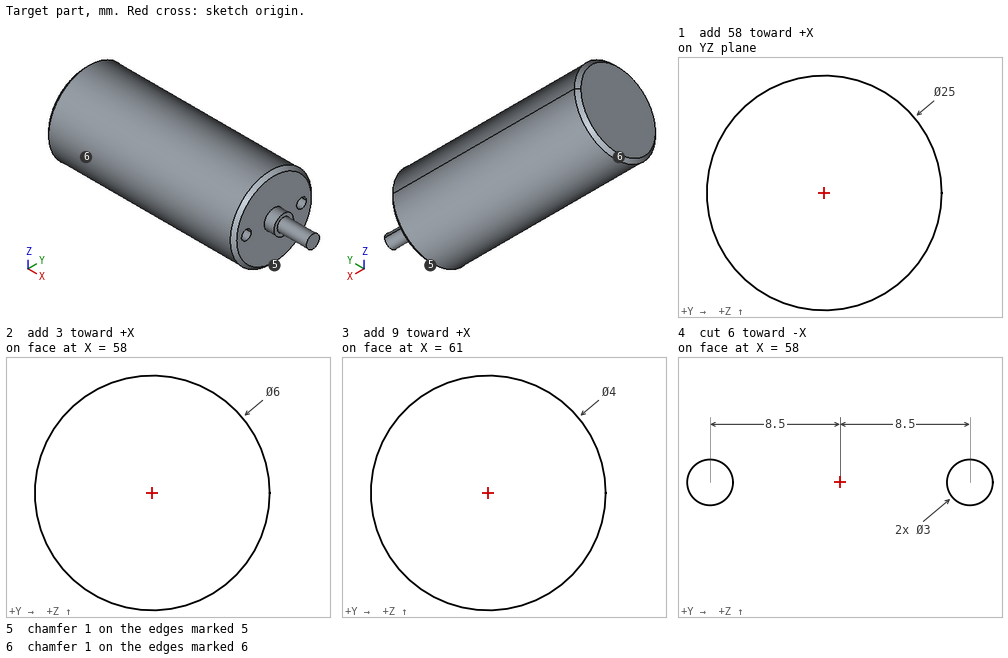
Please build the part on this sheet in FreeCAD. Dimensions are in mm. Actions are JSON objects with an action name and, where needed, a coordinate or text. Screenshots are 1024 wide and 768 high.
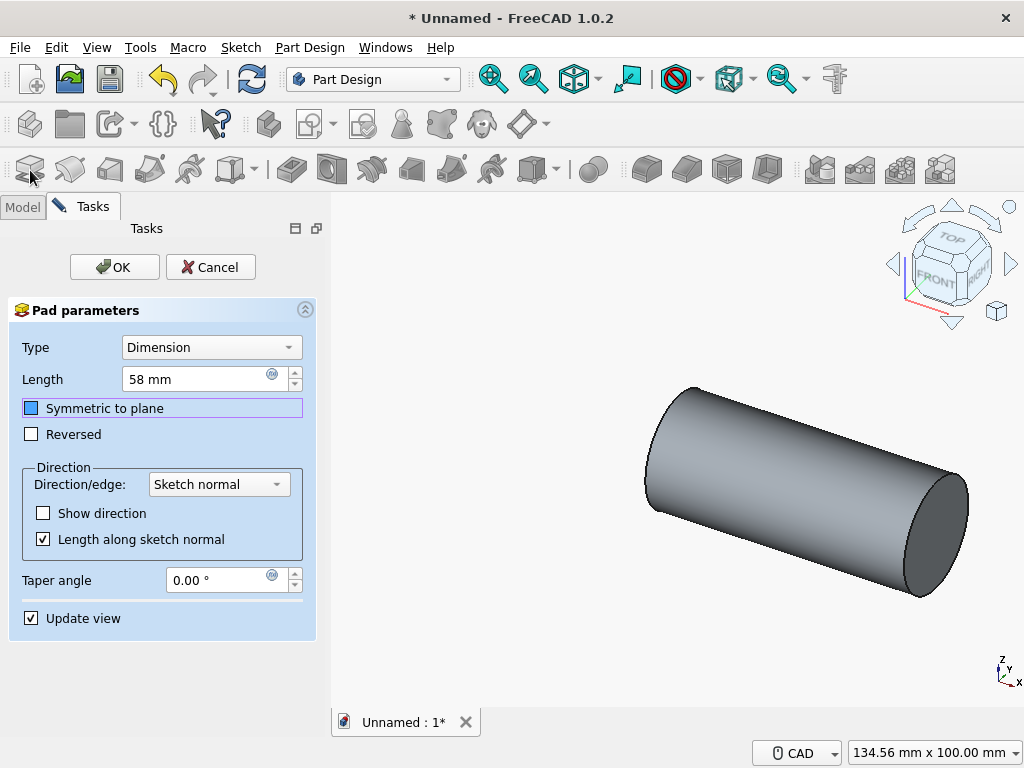
{"action": "left_click", "coordinate": [115, 267]}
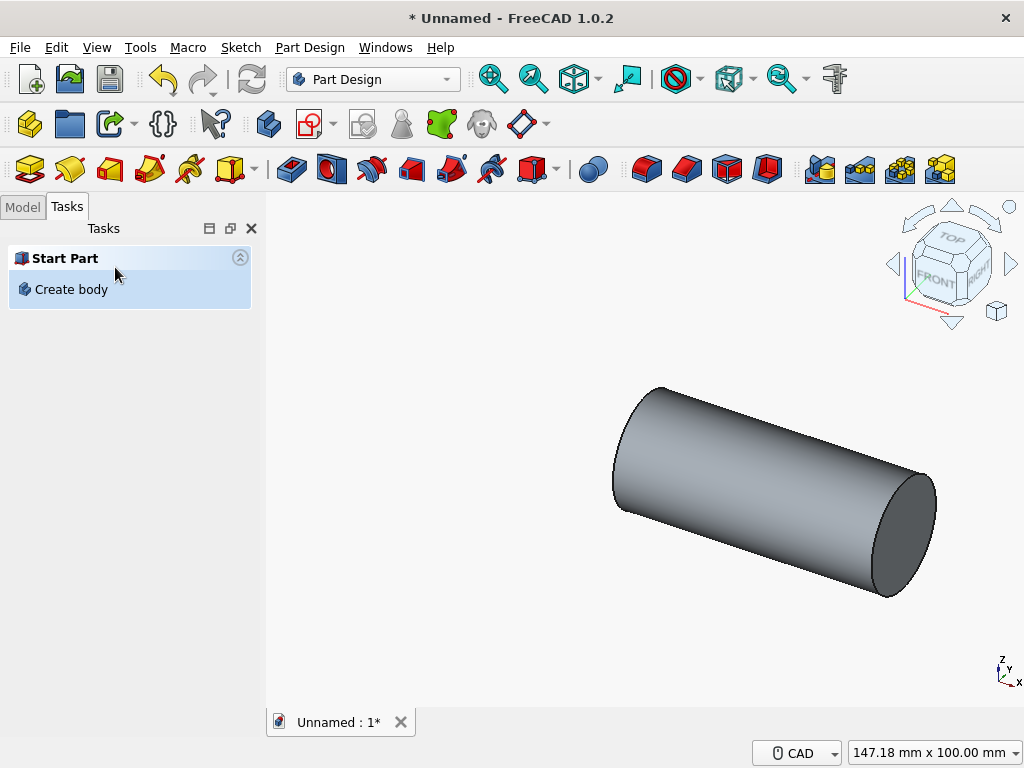
{"action": "left_click", "coordinate": [904, 534]}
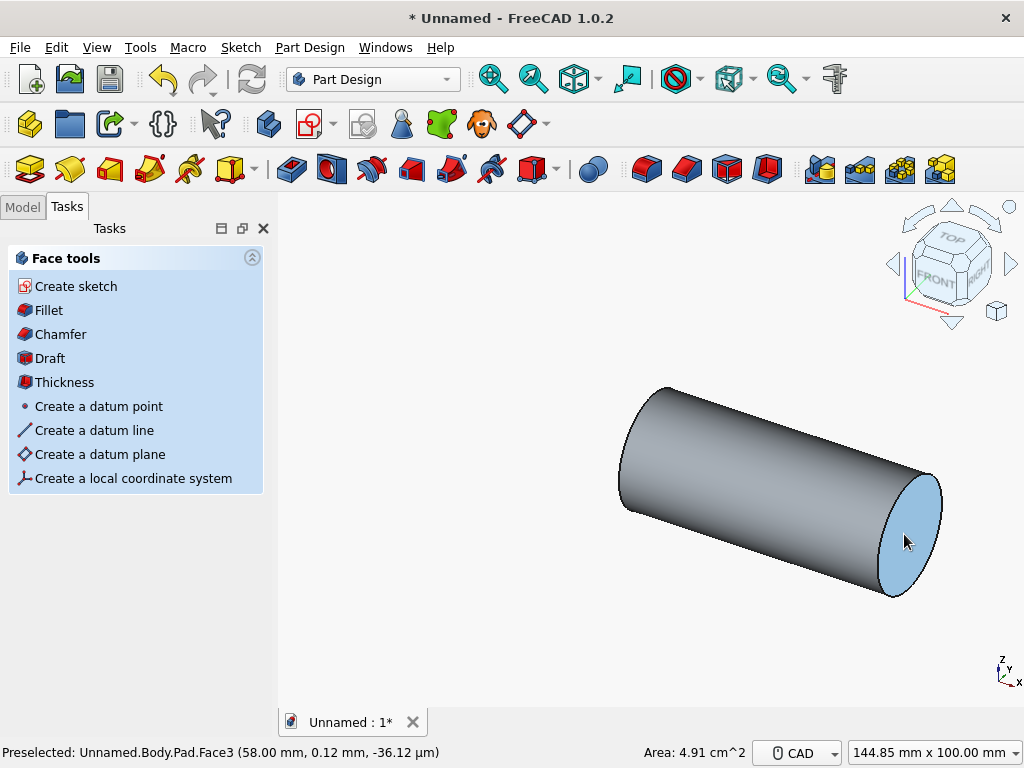
{"action": "left_click", "coordinate": [310, 124]}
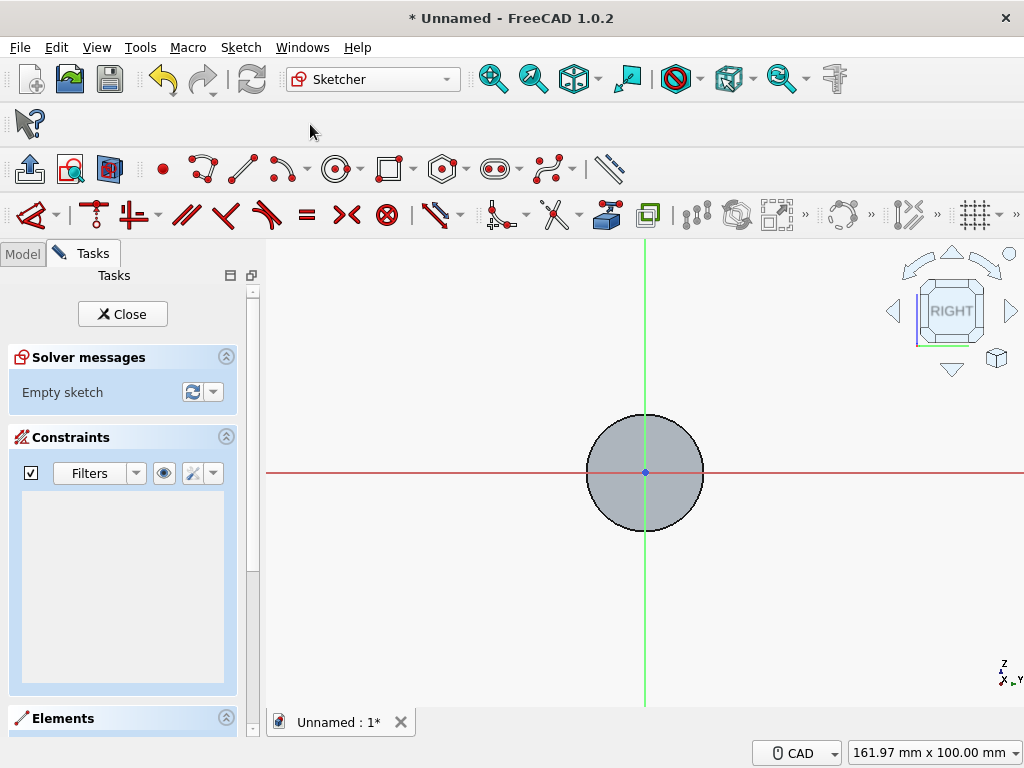
{"action": "scroll", "coordinate": [652, 473], "scroll_direction": "up", "scroll_amount": 12}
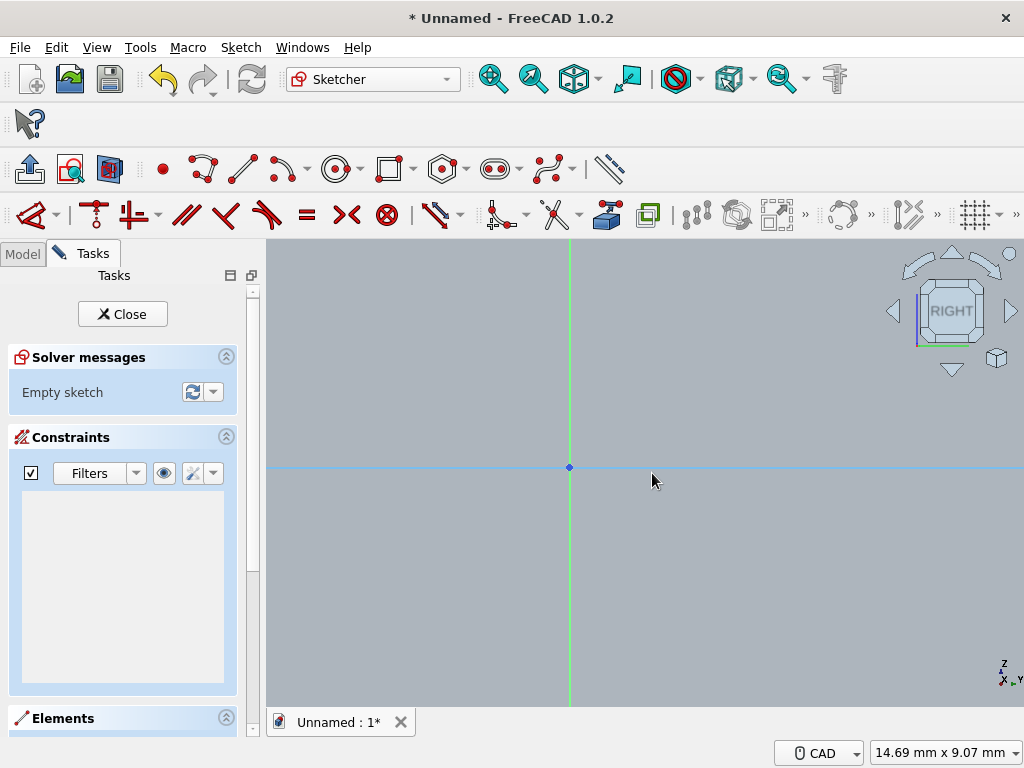
{"action": "left_click", "coordinate": [336, 170]}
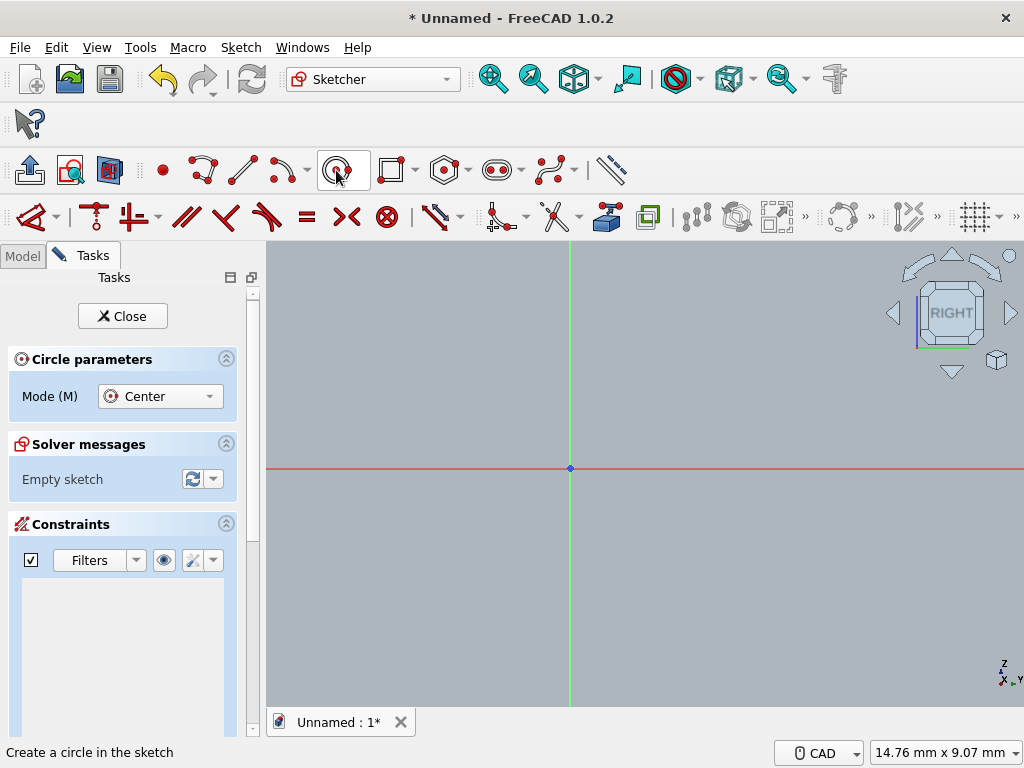
{"action": "left_click", "coordinate": [570, 469]}
{"action": "left_click", "coordinate": [679, 360]}
{"action": "key", "text": "Escape"}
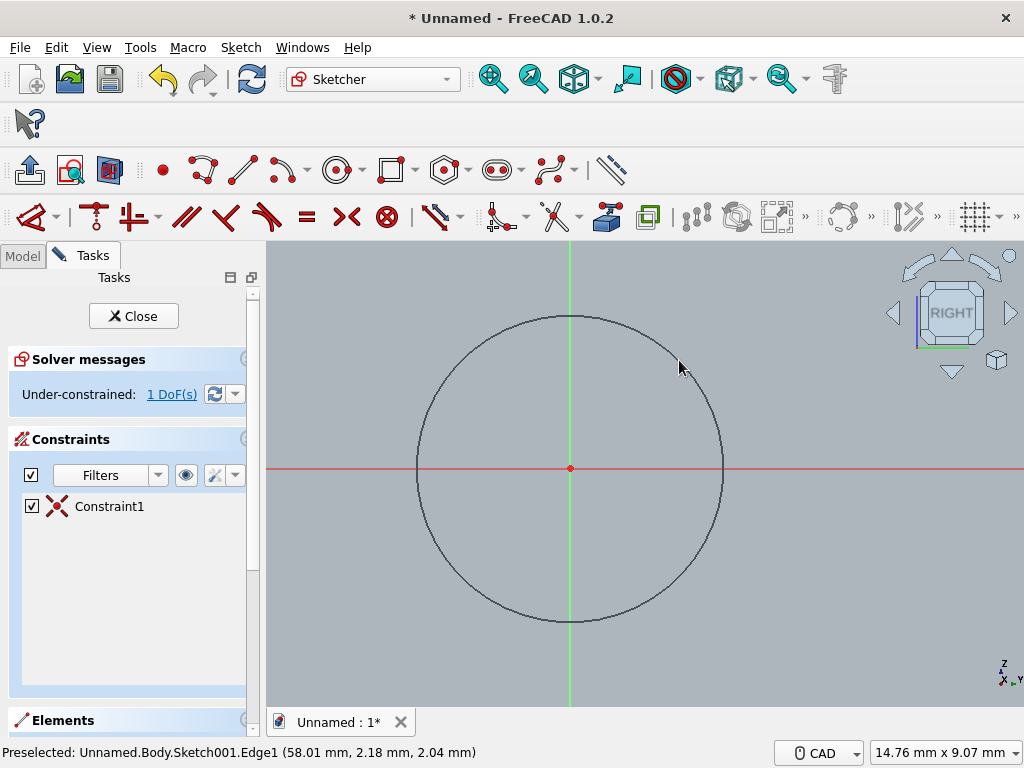
{"action": "left_click", "coordinate": [32, 218]}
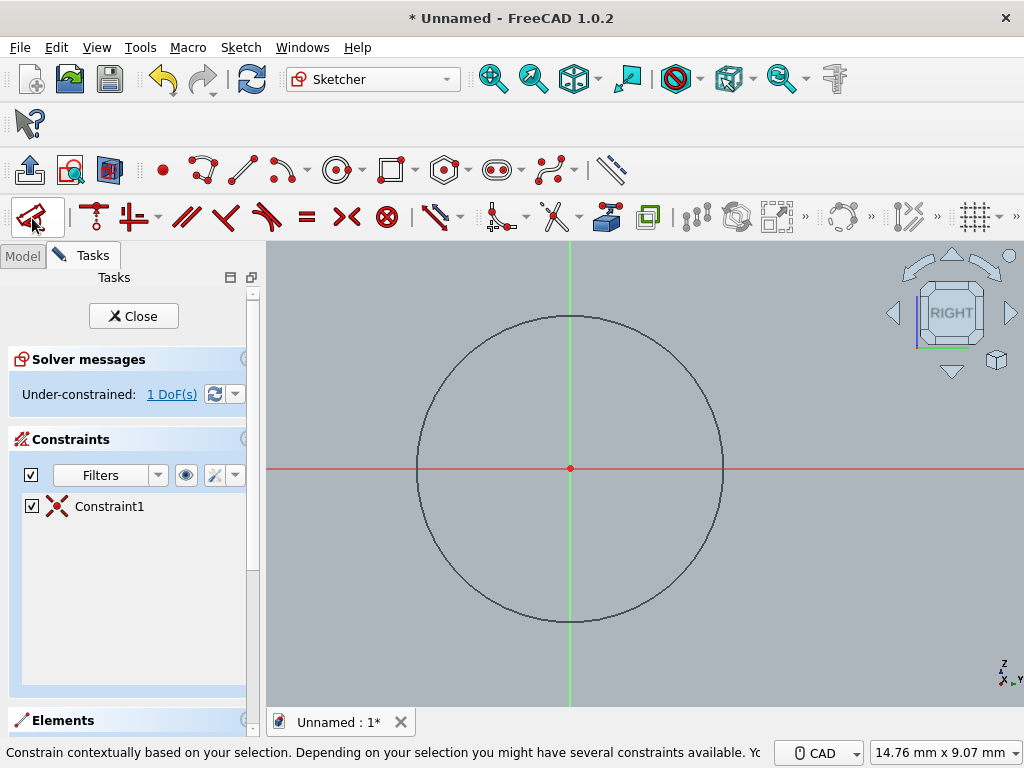
{"action": "left_click", "coordinate": [678, 360]}
{"action": "left_click", "coordinate": [701, 337]}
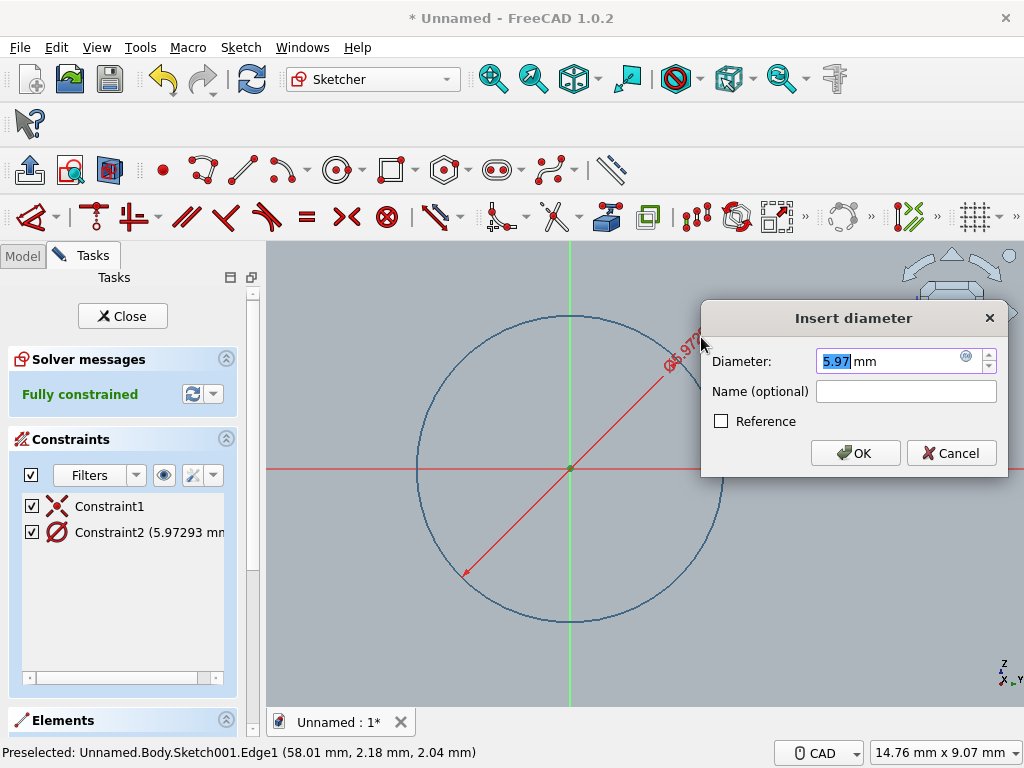
{"action": "type", "text": "6"}
{"action": "key", "text": "Return"}
{"action": "key", "text": "Escape"}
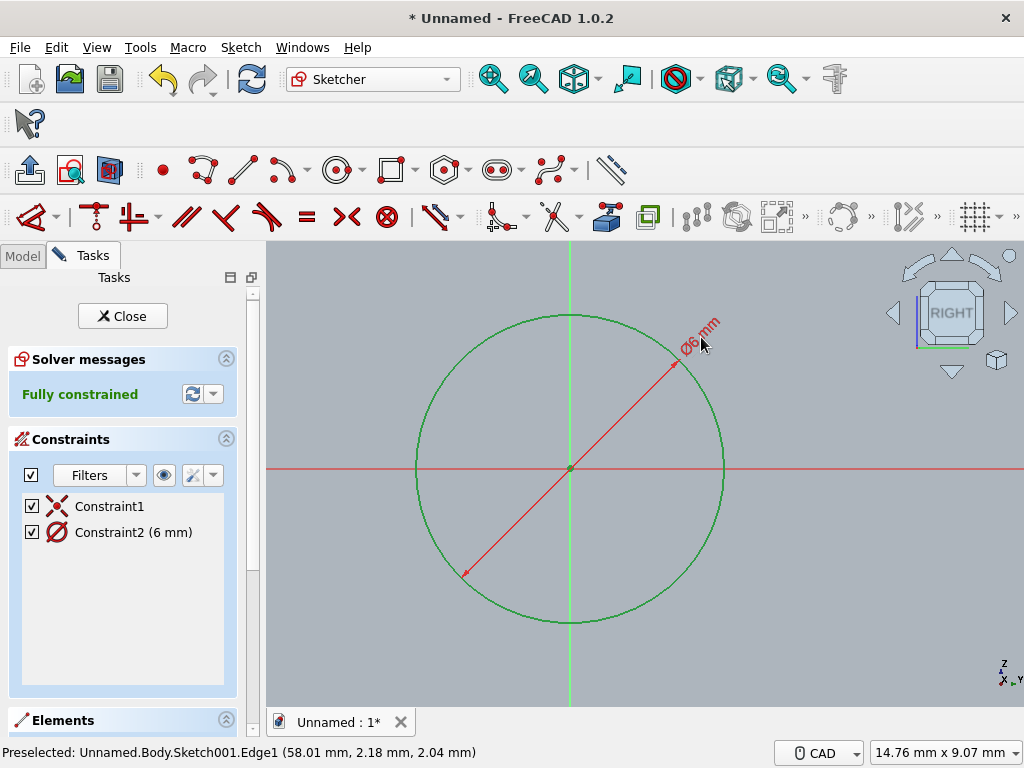
{"action": "left_click", "coordinate": [123, 316]}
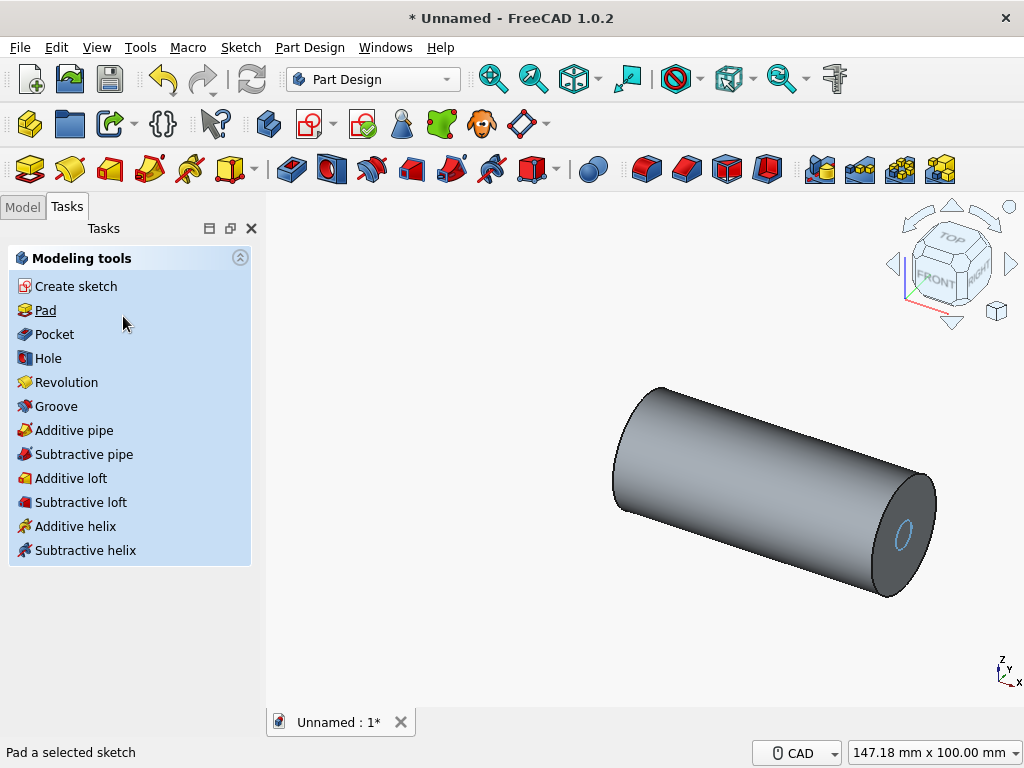
{"action": "left_click", "coordinate": [30, 170]}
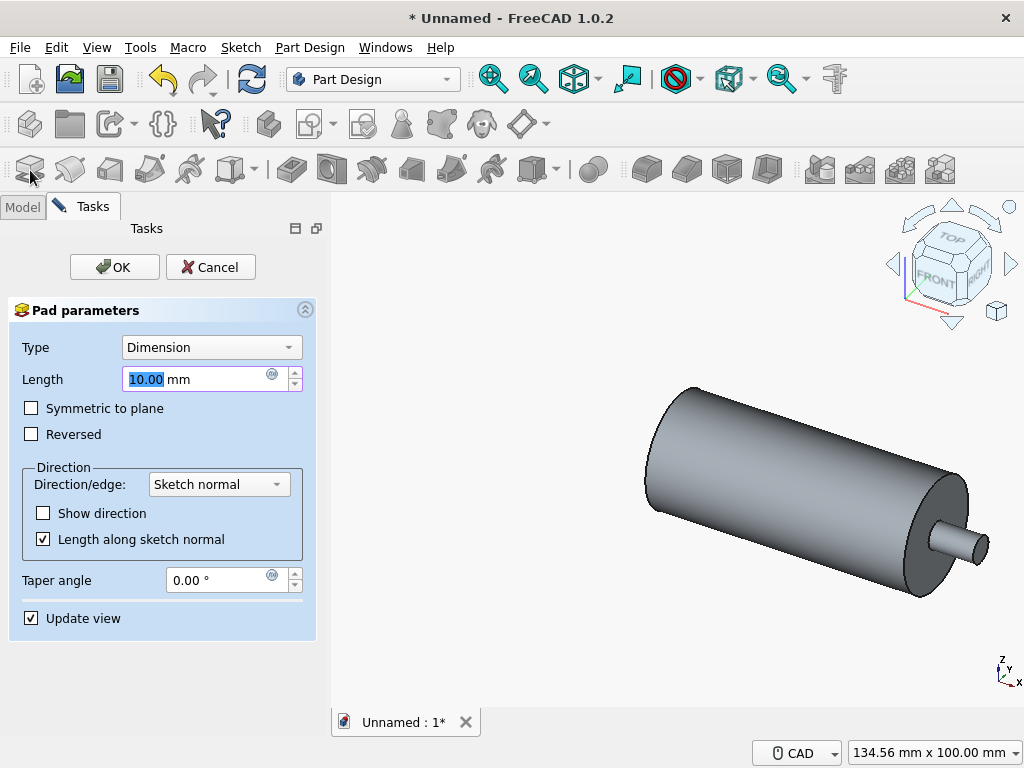
{"action": "type", "text": "3"}
{"action": "key", "text": "Tab"}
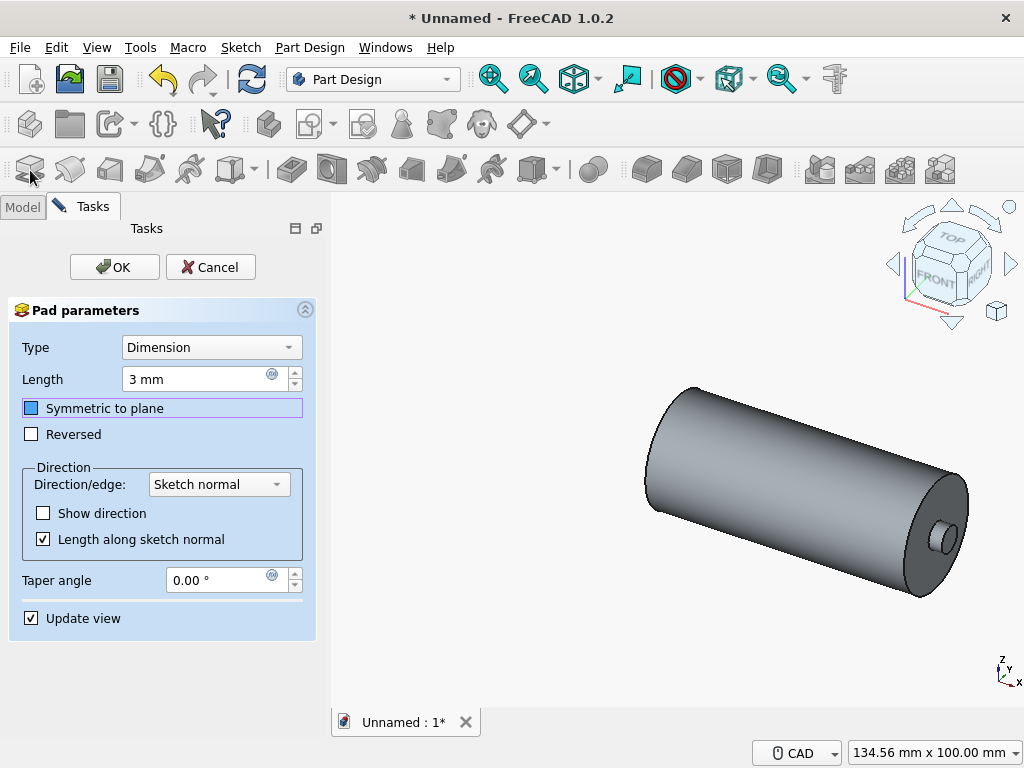
{"action": "left_click", "coordinate": [115, 267]}